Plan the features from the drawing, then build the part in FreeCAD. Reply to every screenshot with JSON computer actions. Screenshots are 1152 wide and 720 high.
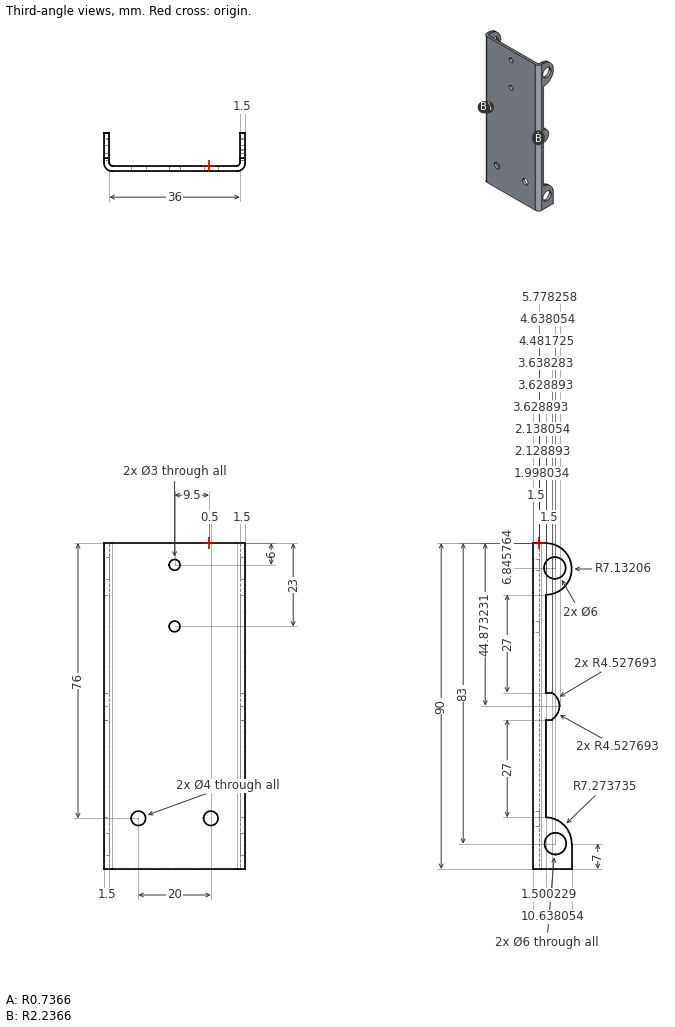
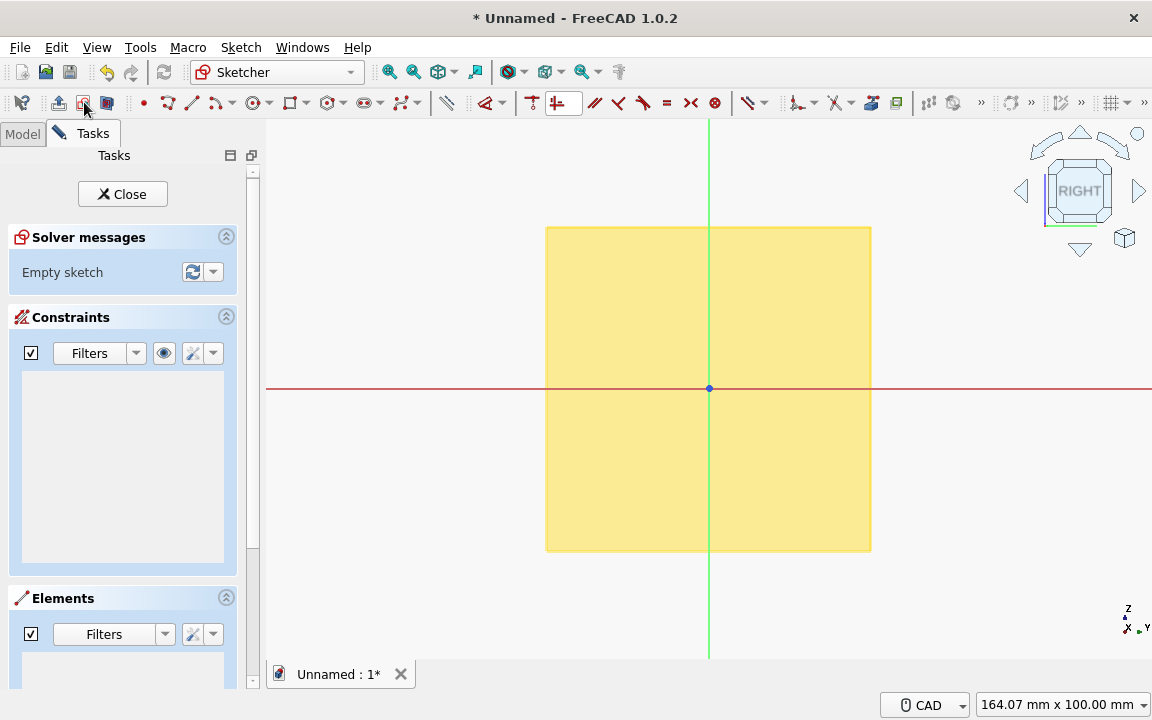
{"action": "scroll", "coordinate": [532, 147], "scroll_direction": "down", "scroll_amount": 3}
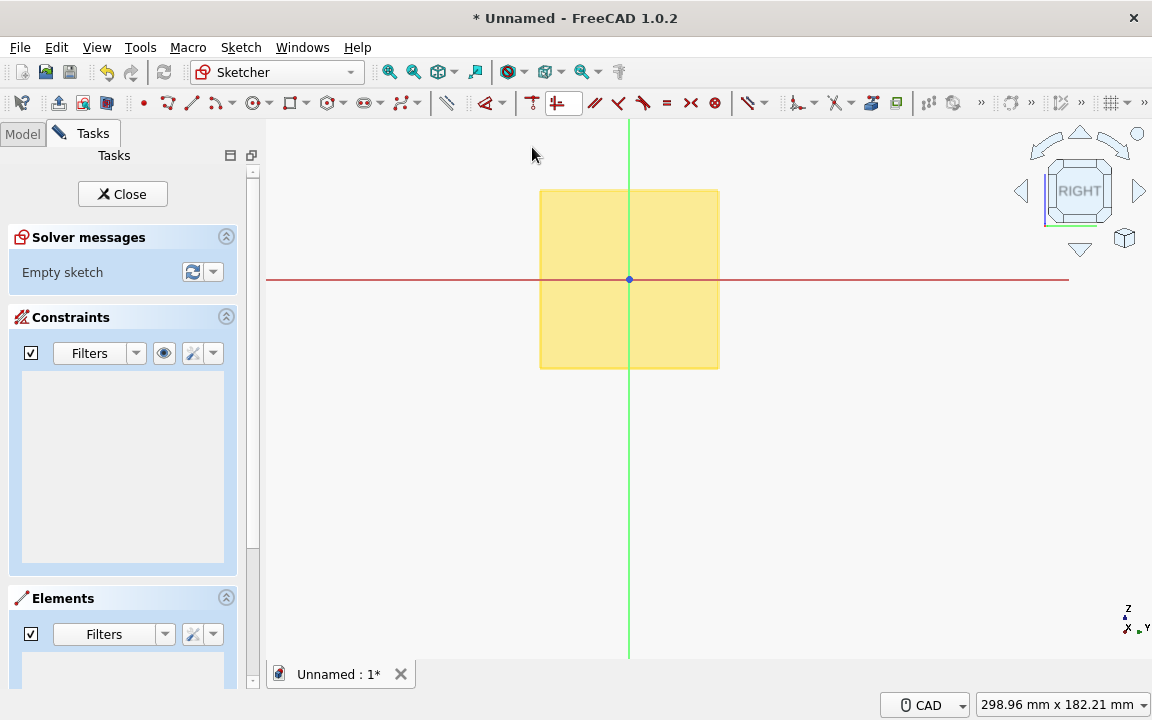
{"action": "key", "text": "g m"}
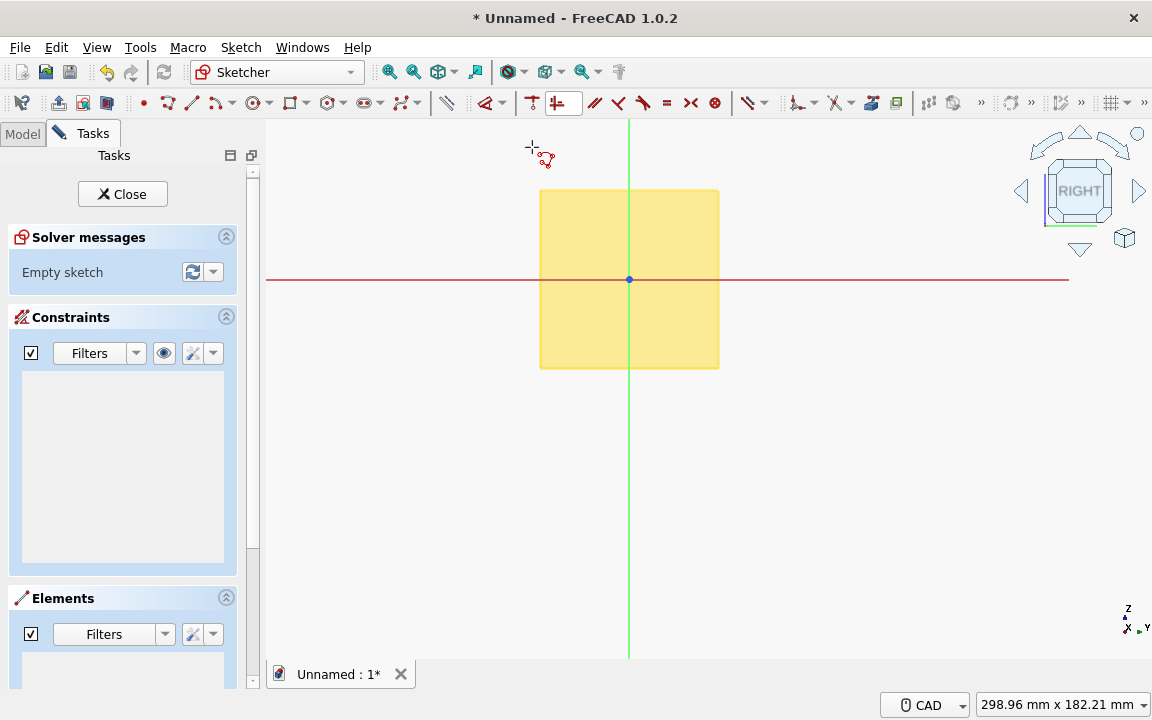
{"action": "scroll", "coordinate": [636, 322], "scroll_direction": "up", "scroll_amount": 5}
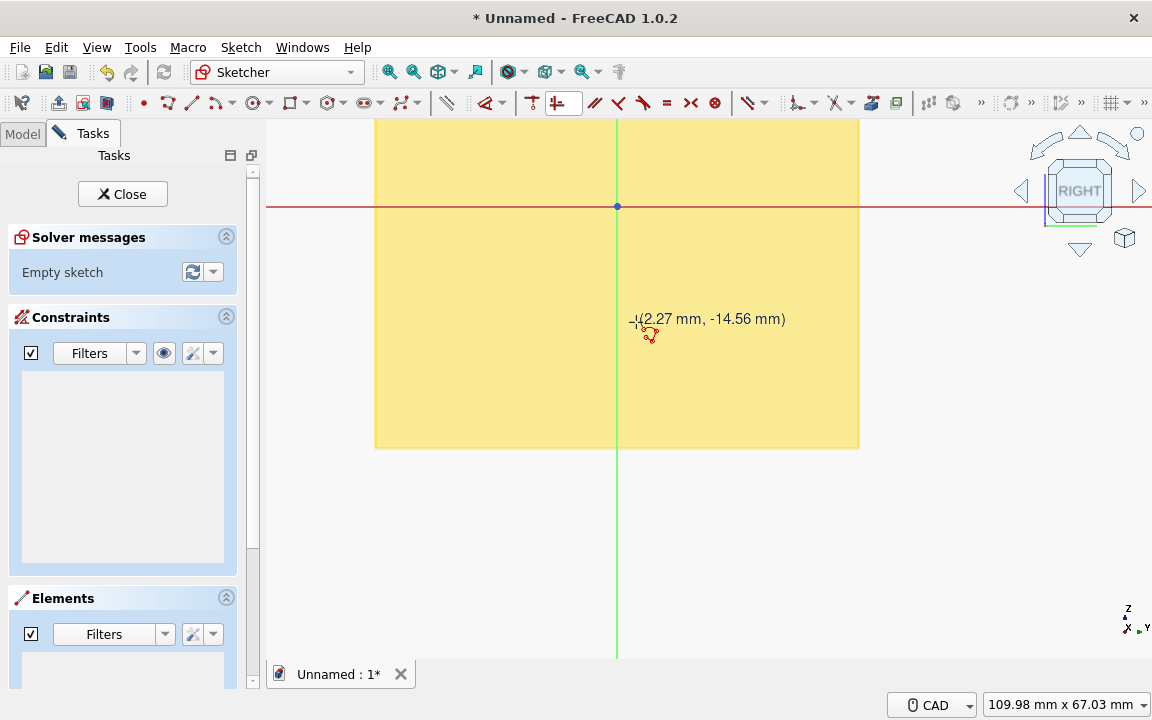
{"action": "left_click", "coordinate": [634, 322]}
{"action": "left_click", "coordinate": [634, 539]}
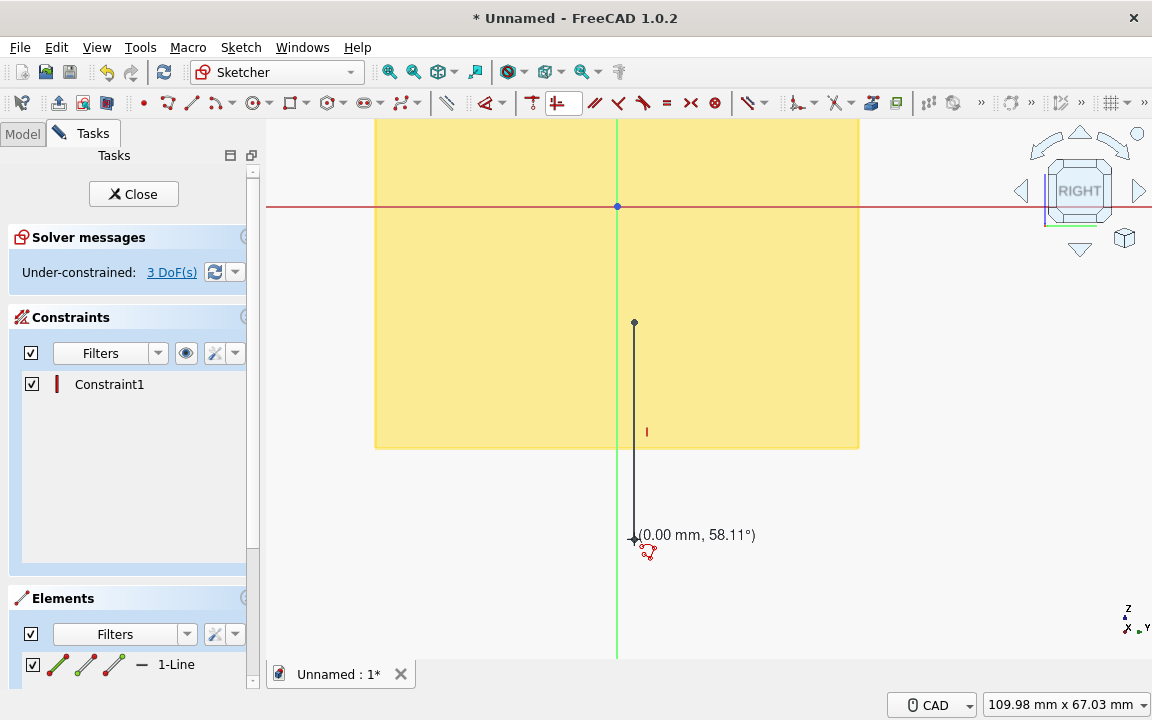
{"action": "scroll", "coordinate": [646, 539], "scroll_direction": "up", "scroll_amount": 2}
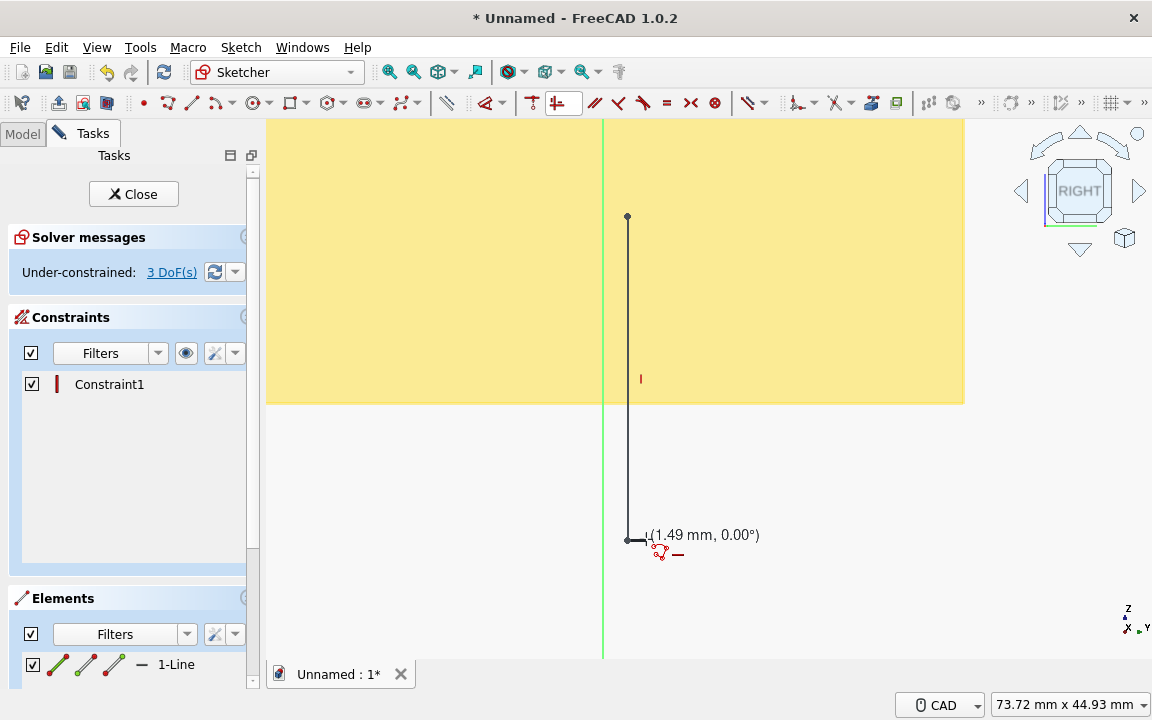
{"action": "left_click", "coordinate": [646, 539]}
{"action": "right_click", "coordinate": [646, 539]}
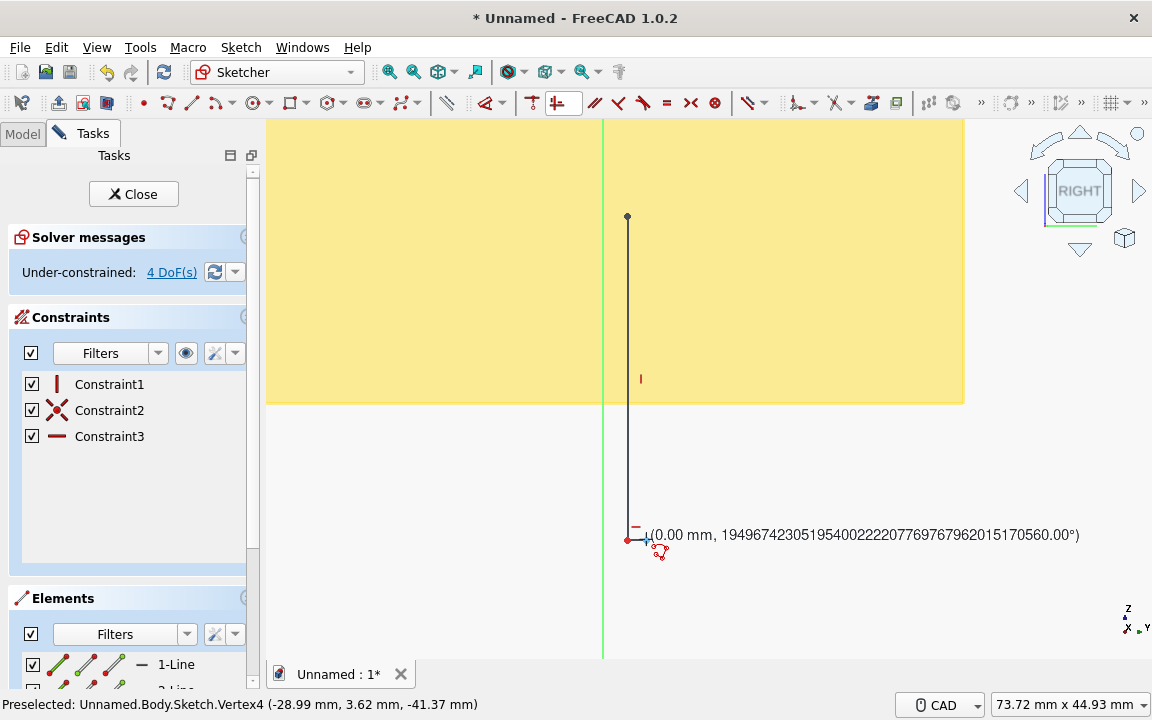
{"action": "left_click", "coordinate": [646, 629]}
{"action": "left_click", "coordinate": [628, 629]}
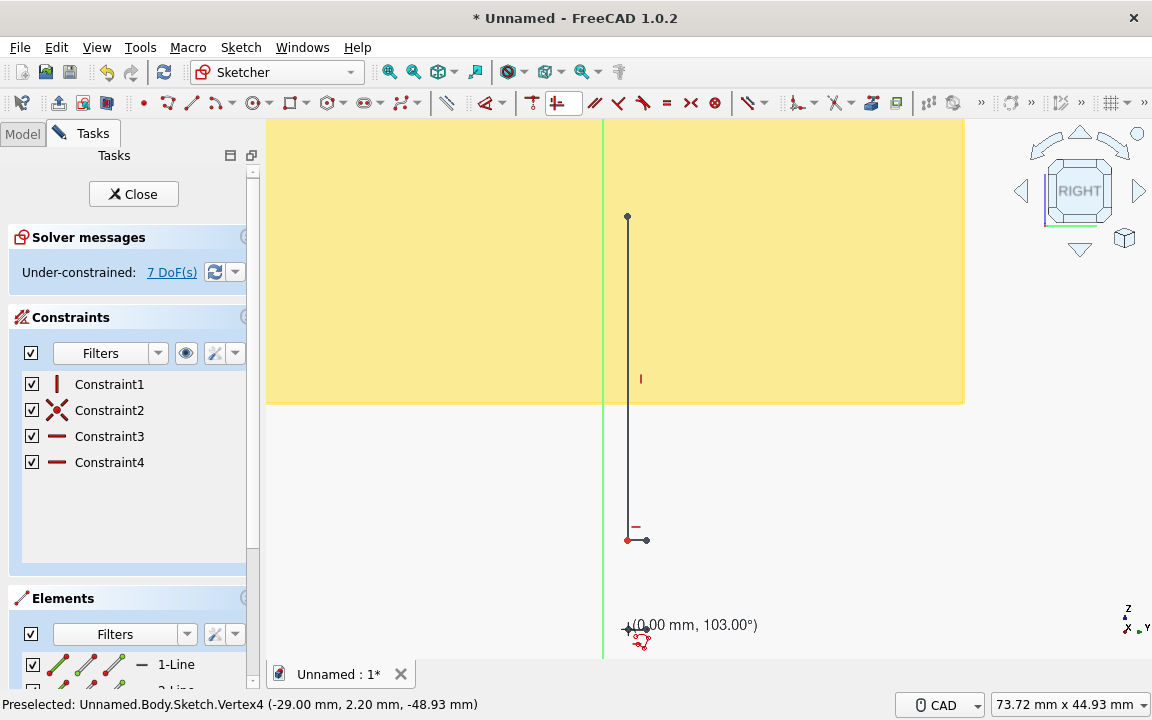
{"action": "scroll", "coordinate": [637, 305], "scroll_direction": "down", "scroll_amount": 6}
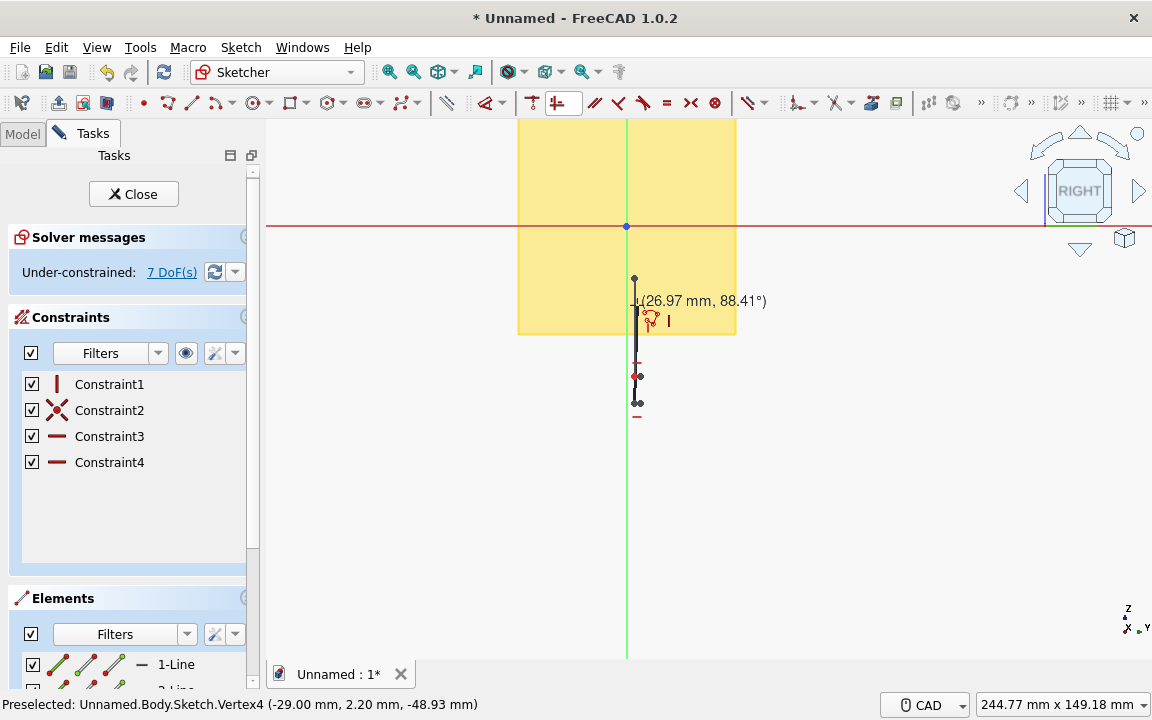
{"action": "scroll", "coordinate": [635, 500], "scroll_direction": "up", "scroll_amount": 4}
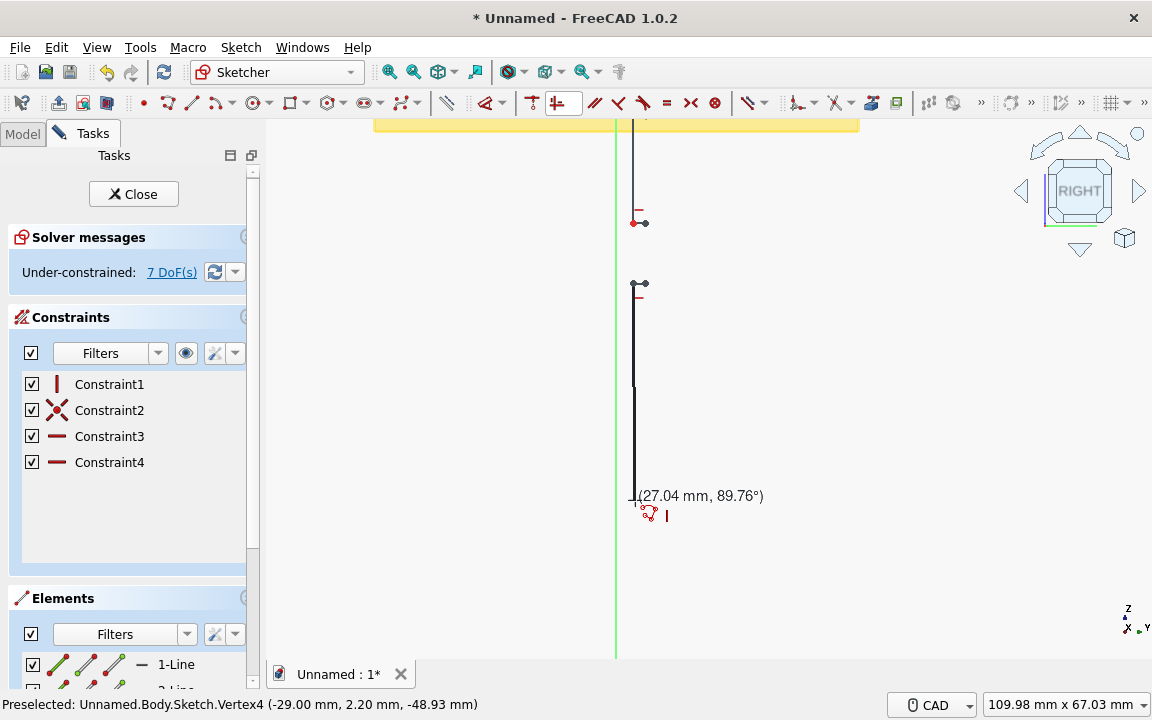
{"action": "left_click", "coordinate": [634, 500]}
{"action": "right_click", "coordinate": [634, 500]}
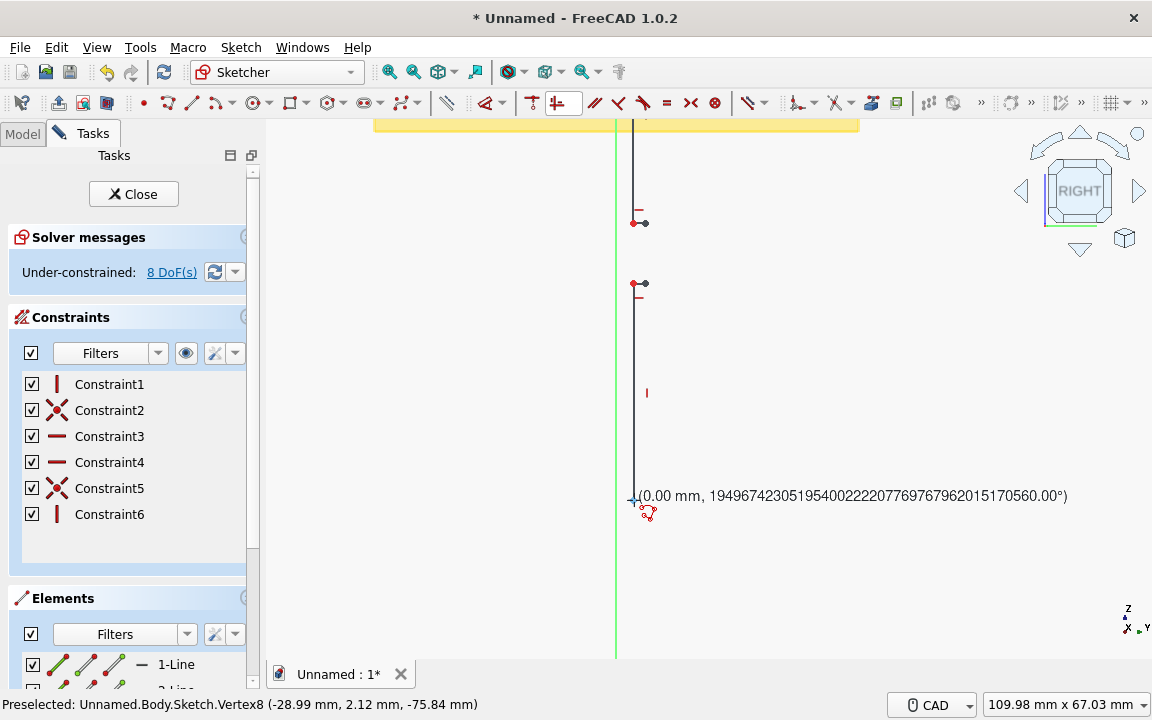
{"action": "left_click", "coordinate": [690, 559]}
{"action": "left_click", "coordinate": [690, 615]}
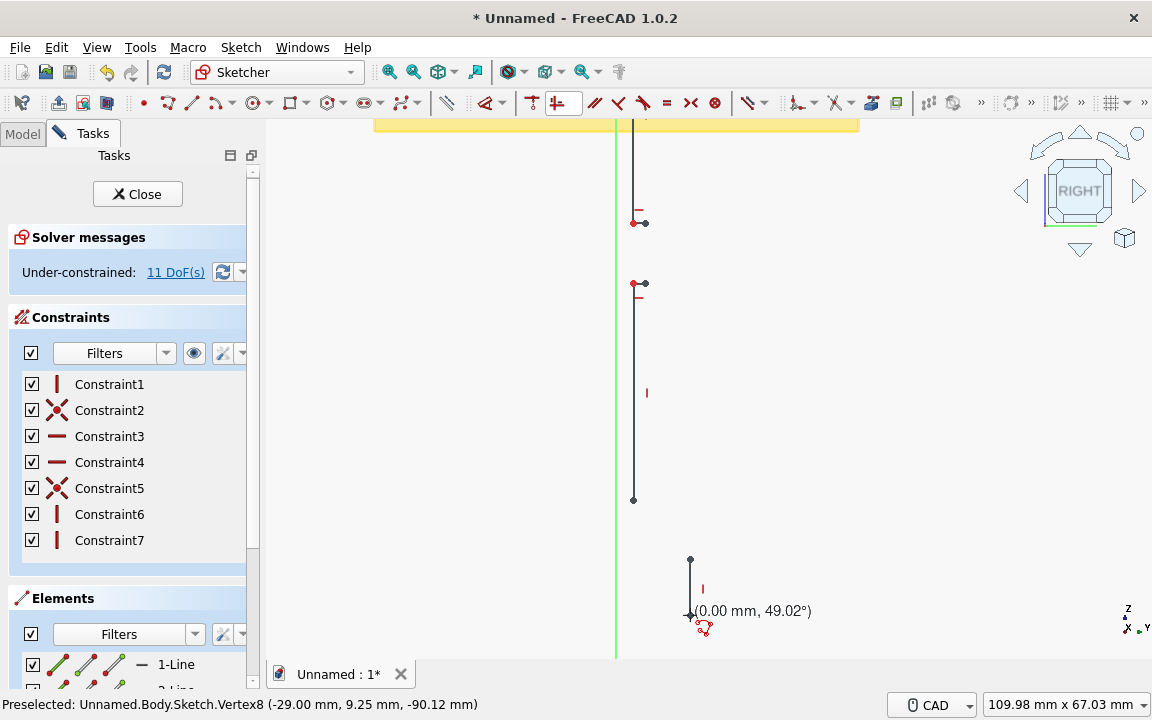
{"action": "scroll", "coordinate": [604, 615], "scroll_direction": "up", "scroll_amount": 2}